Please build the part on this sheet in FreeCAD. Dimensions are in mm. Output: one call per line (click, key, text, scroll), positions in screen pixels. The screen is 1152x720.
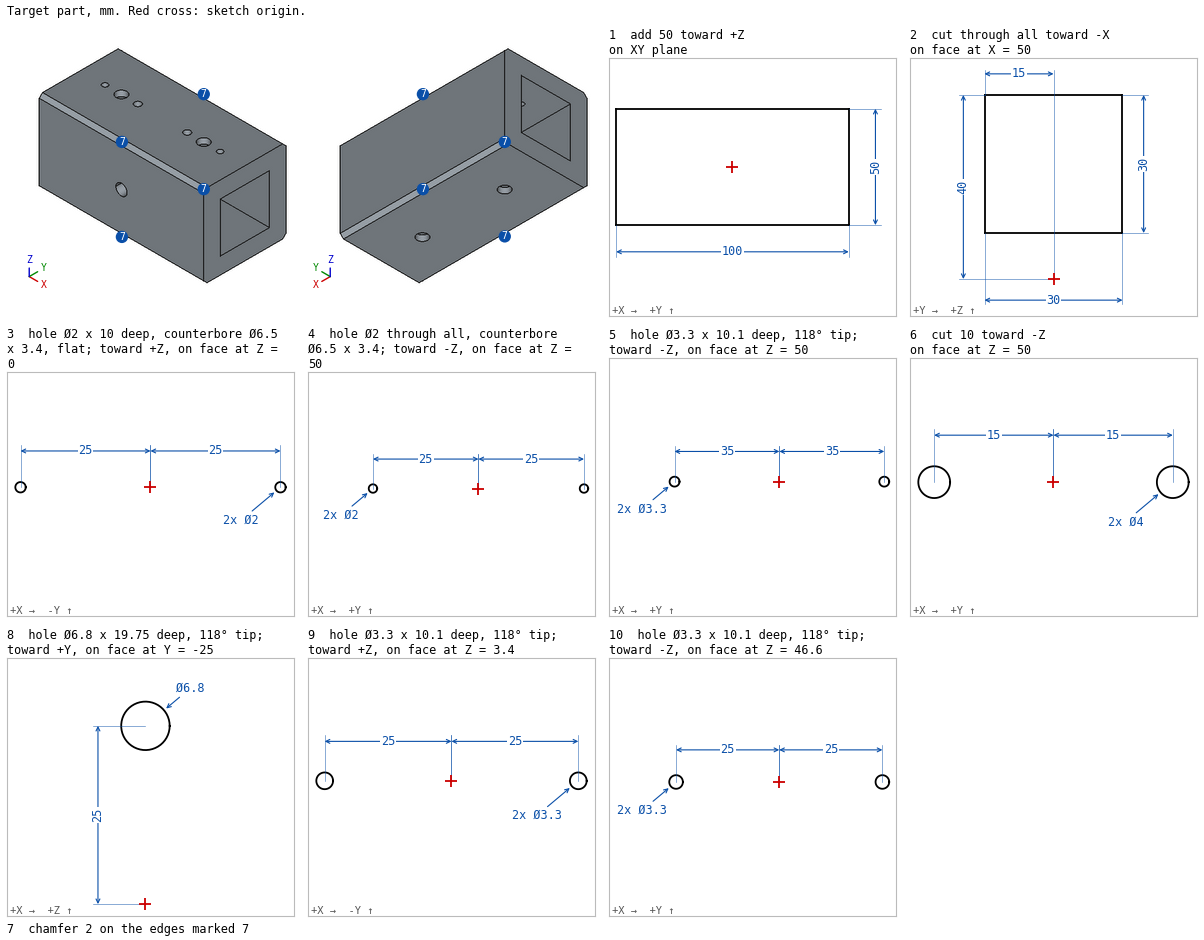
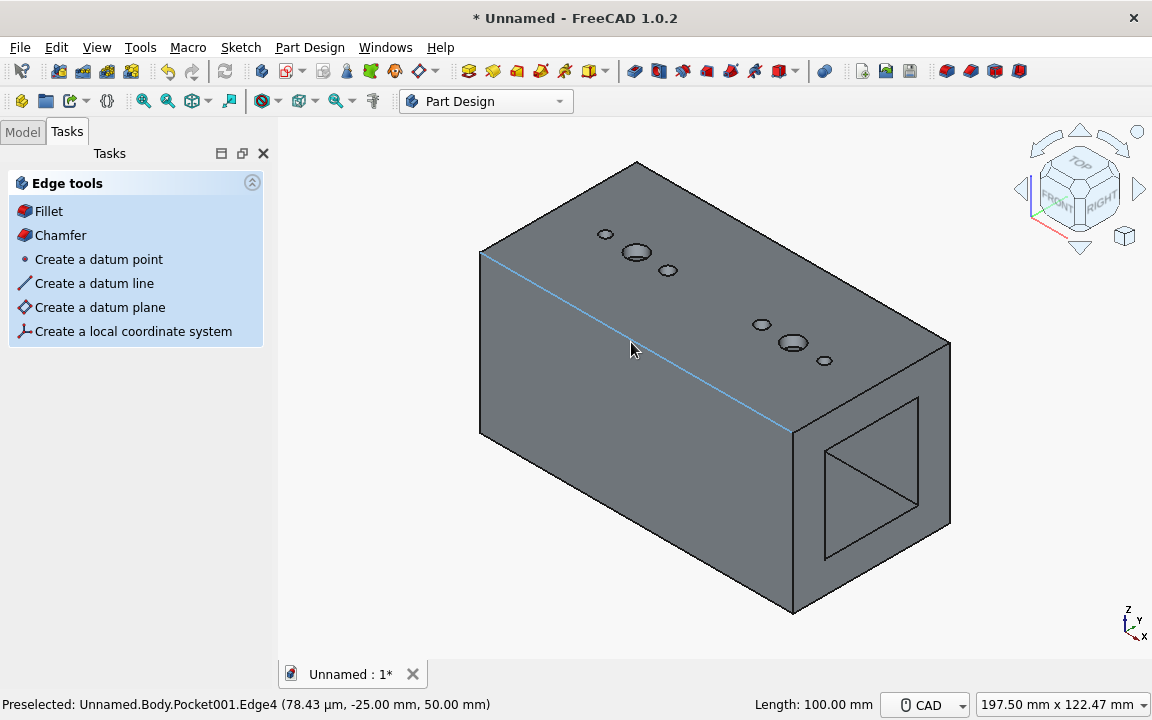
key(2)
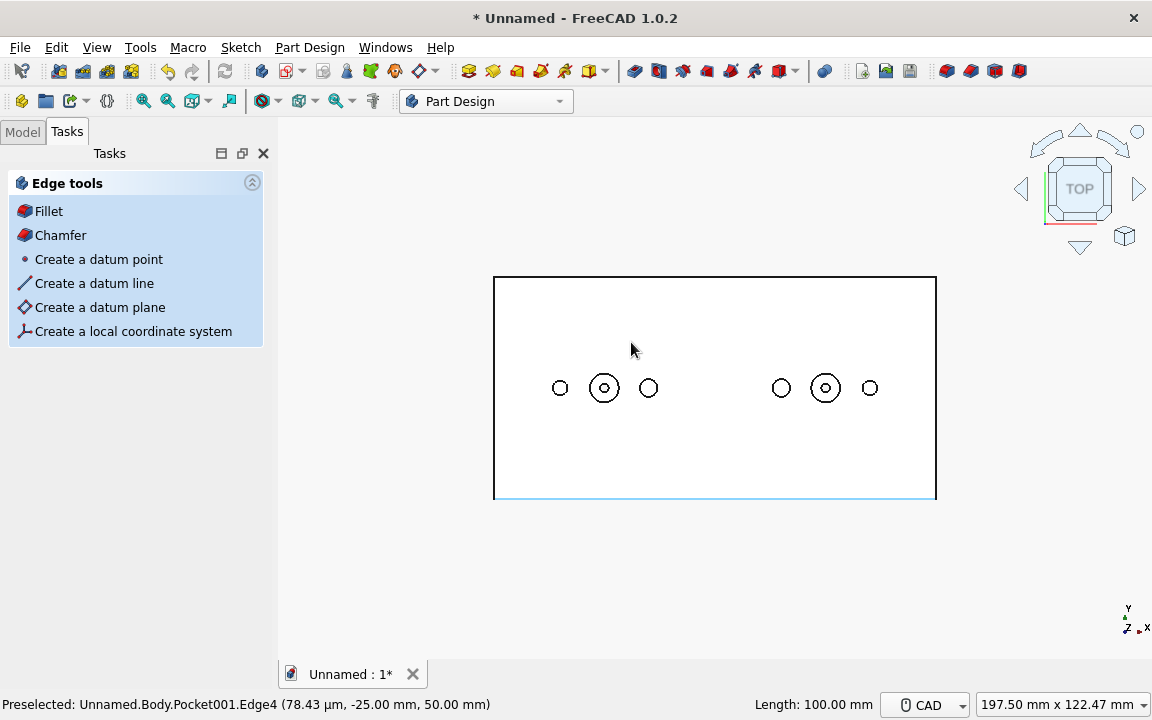
click(715, 276, ctrl)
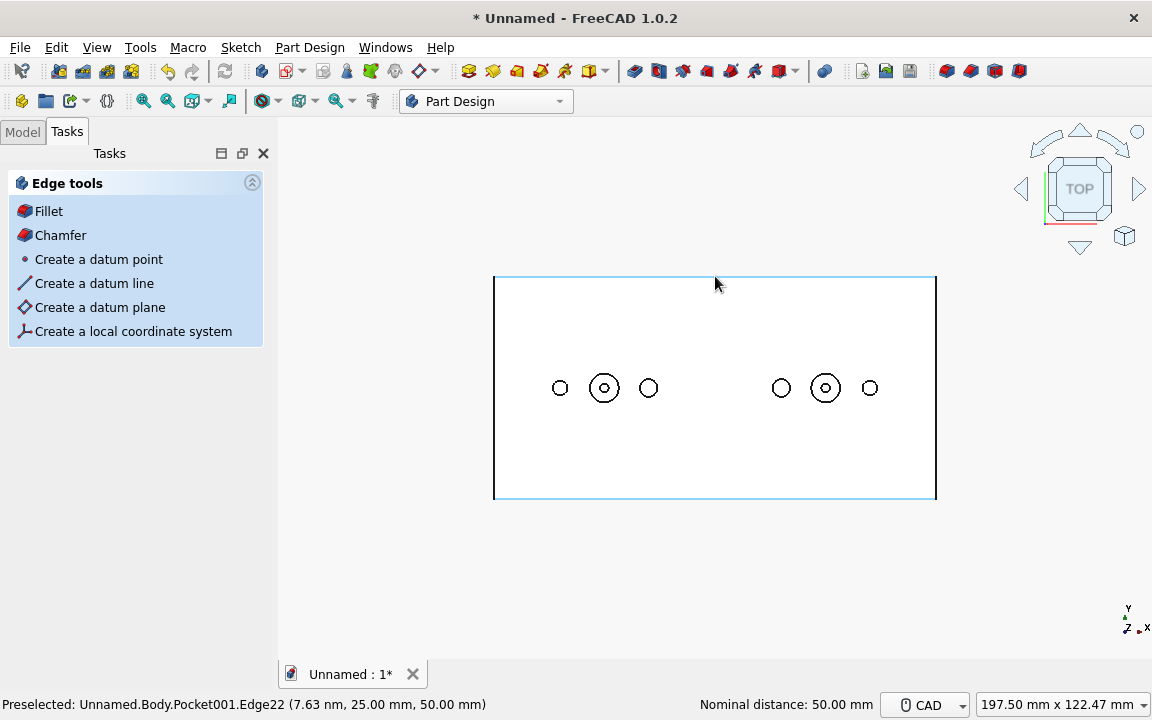
key(0)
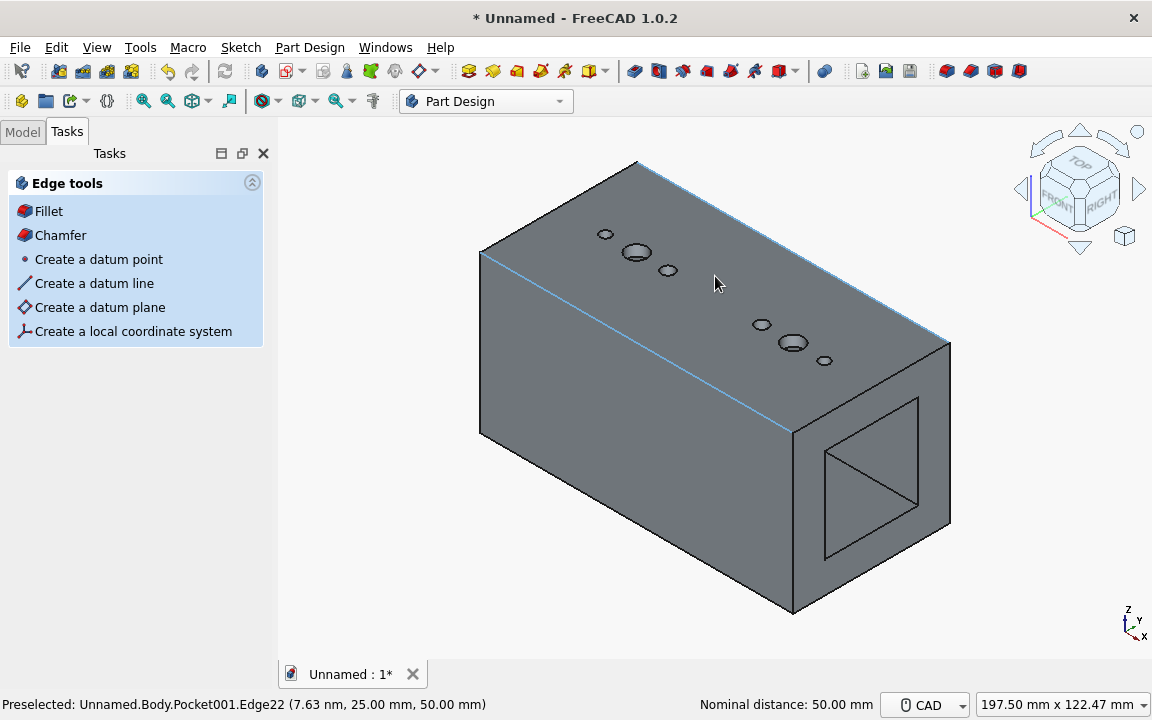
key(1)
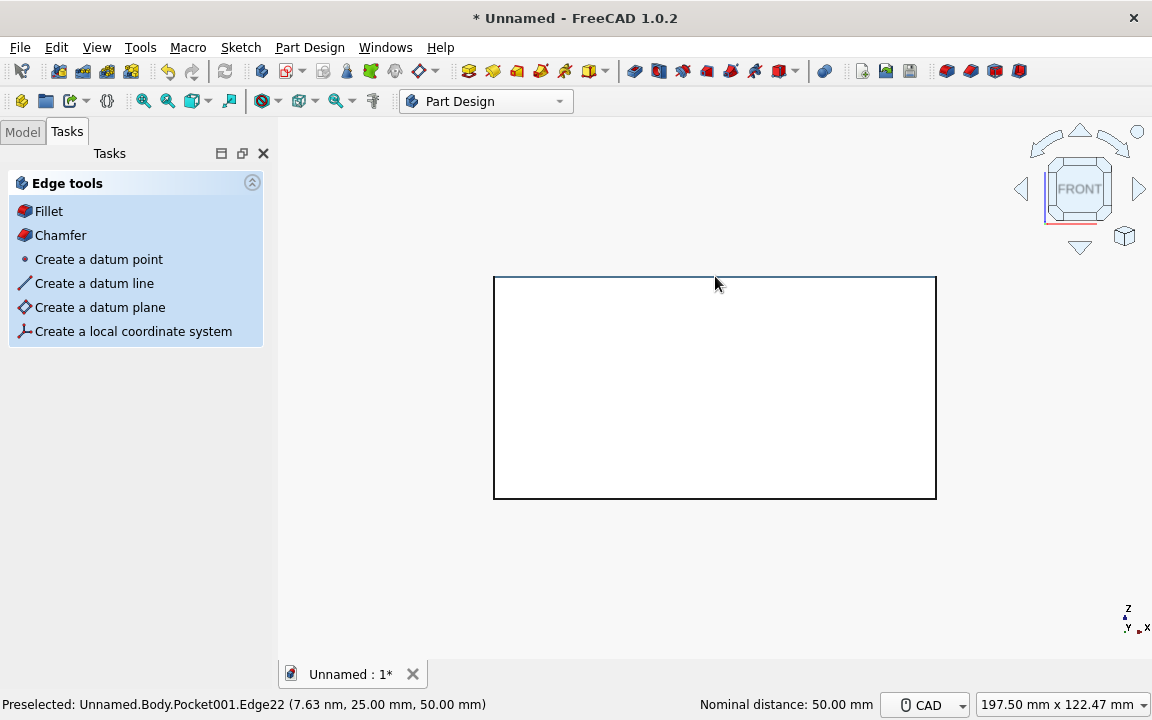
click(715, 498, ctrl)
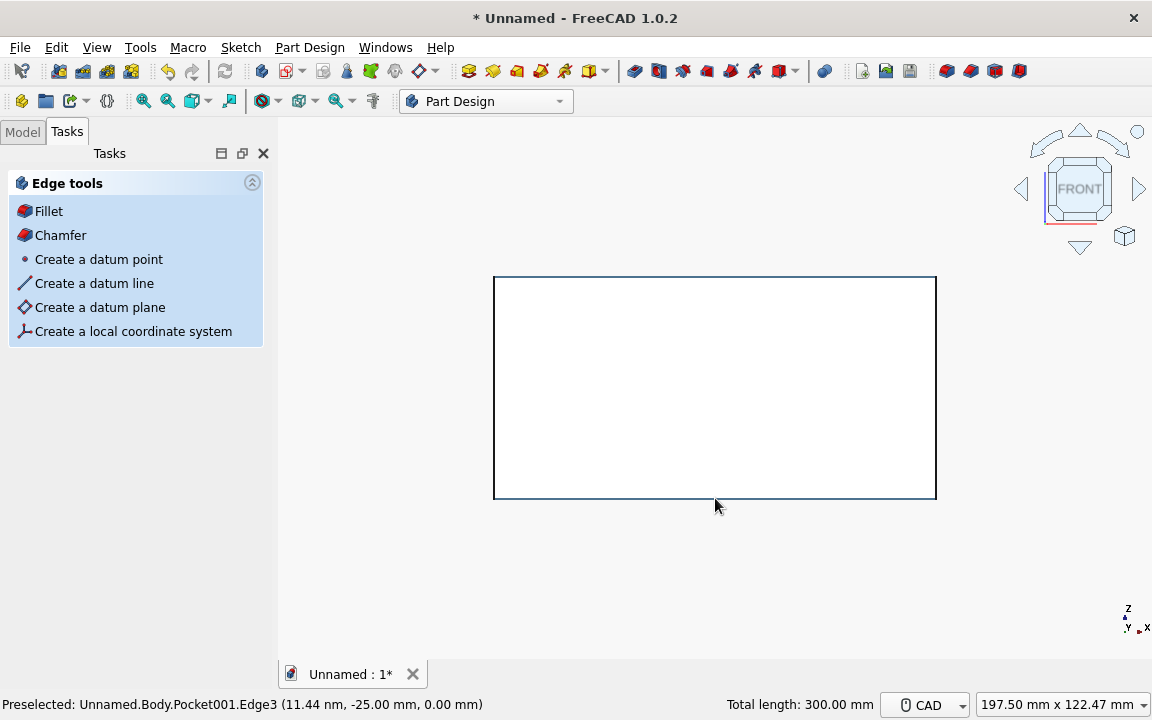
key(3)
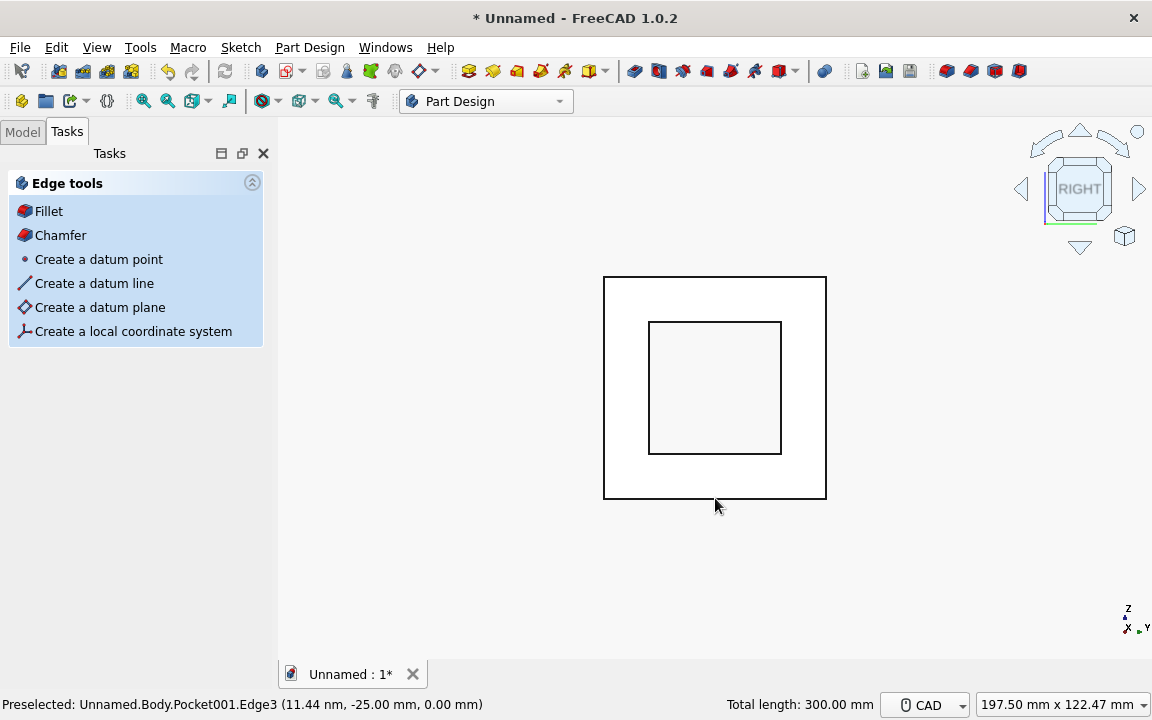
click(144, 102)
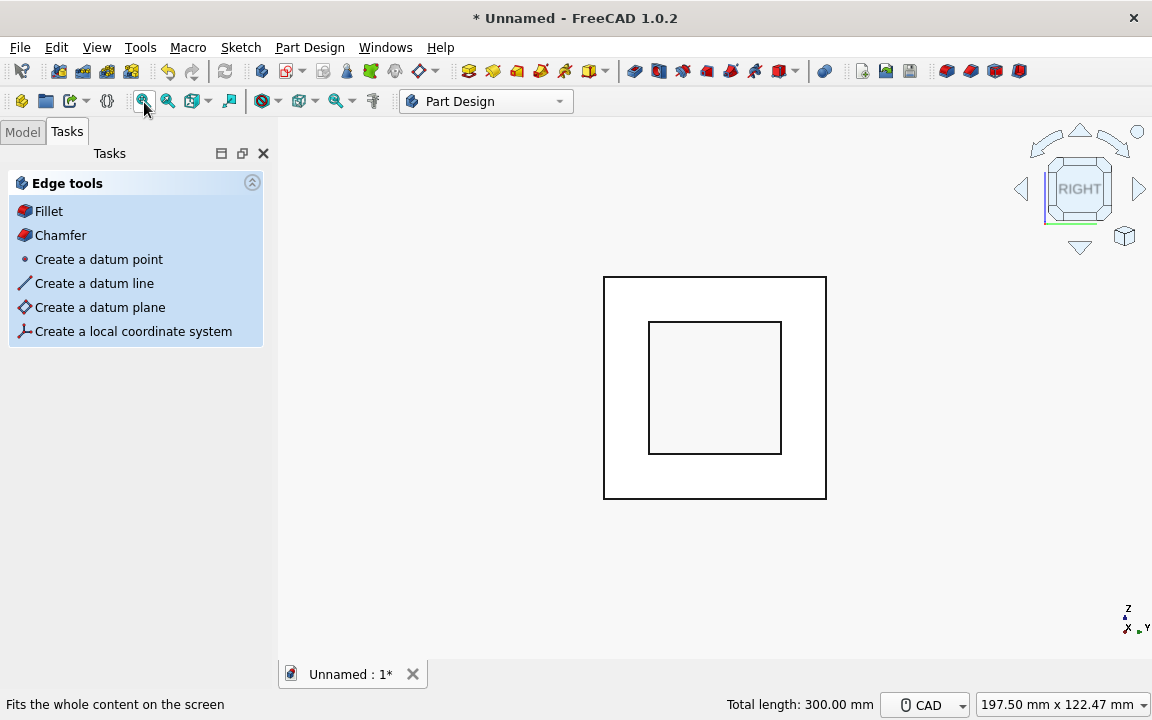
key(5)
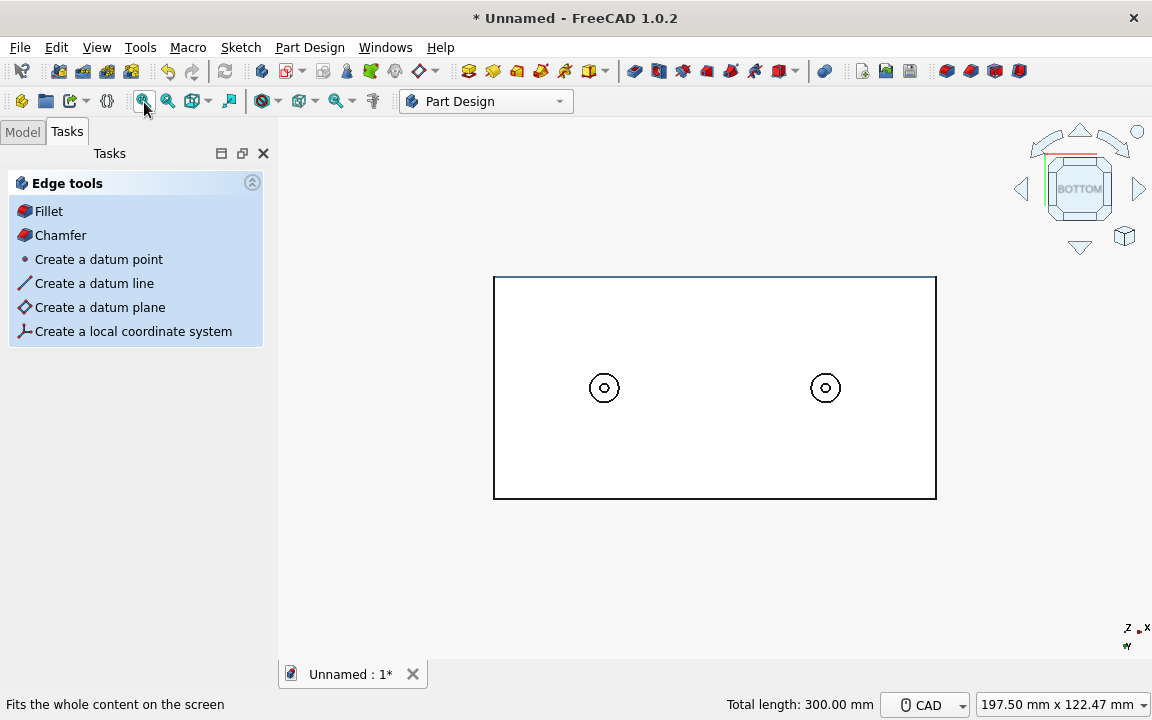
click(715, 498, ctrl)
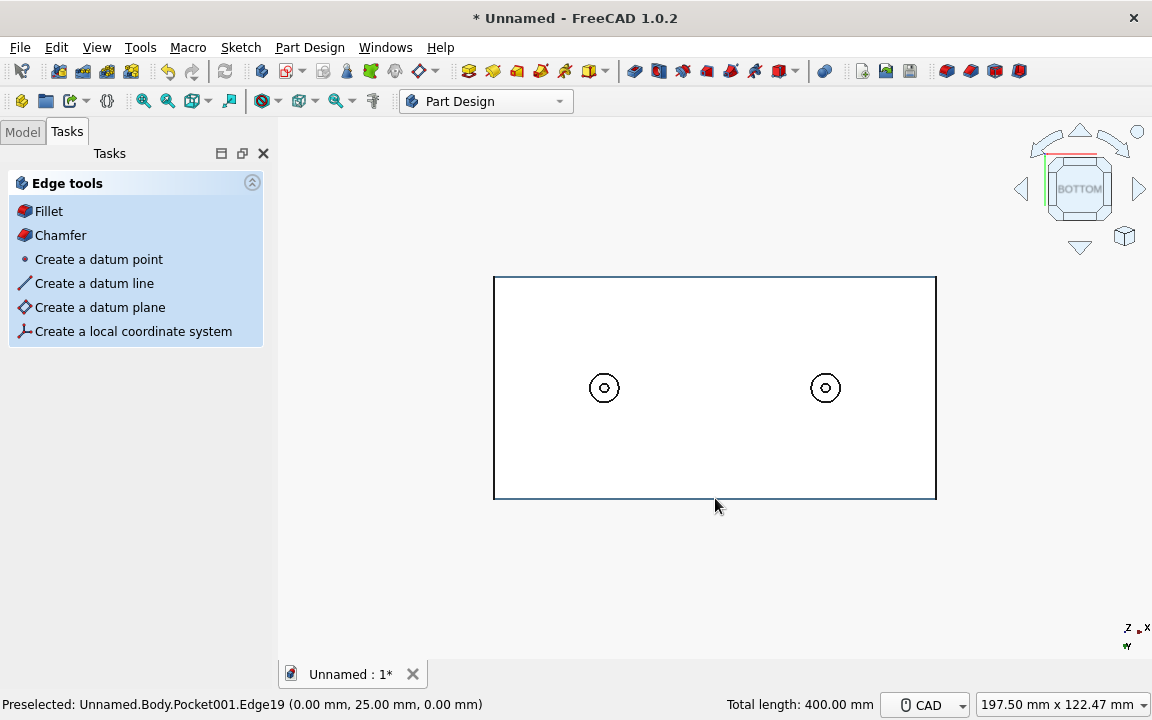
click(972, 72)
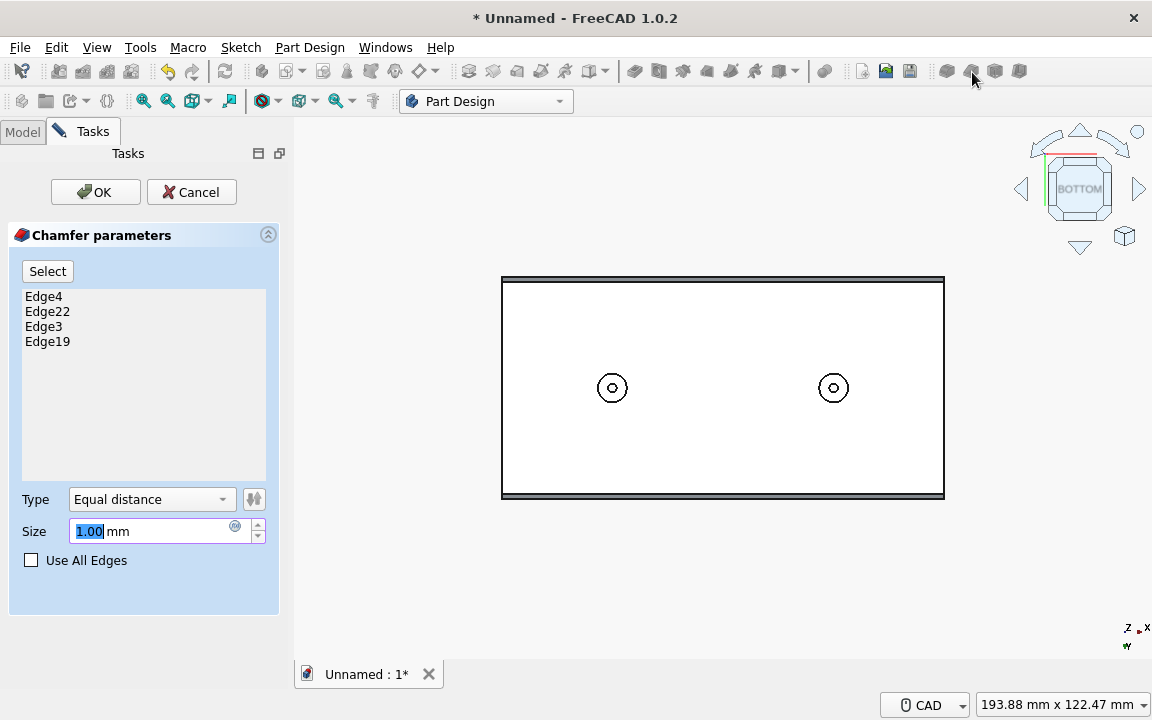
text(2)
key(Tab)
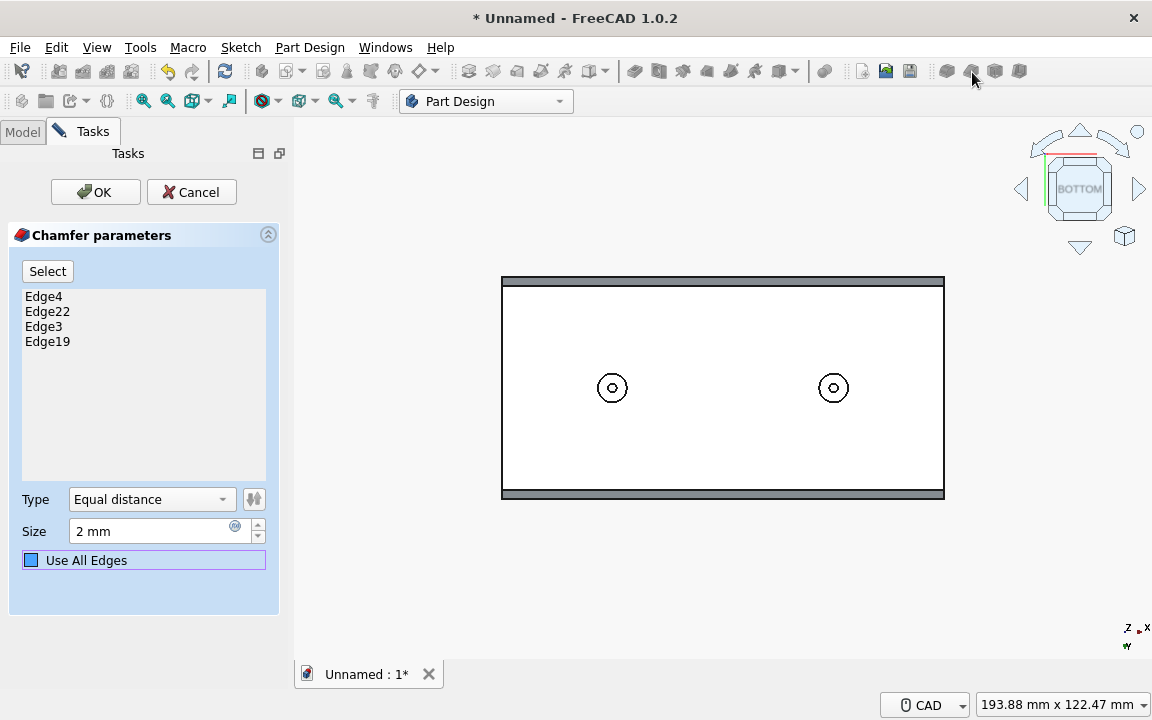
click(96, 192)